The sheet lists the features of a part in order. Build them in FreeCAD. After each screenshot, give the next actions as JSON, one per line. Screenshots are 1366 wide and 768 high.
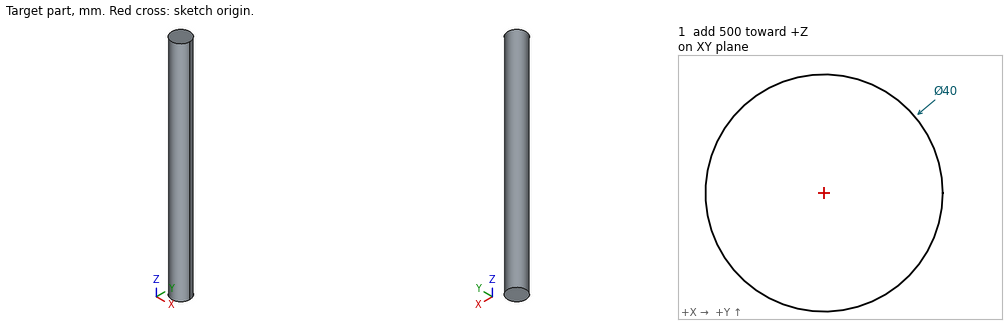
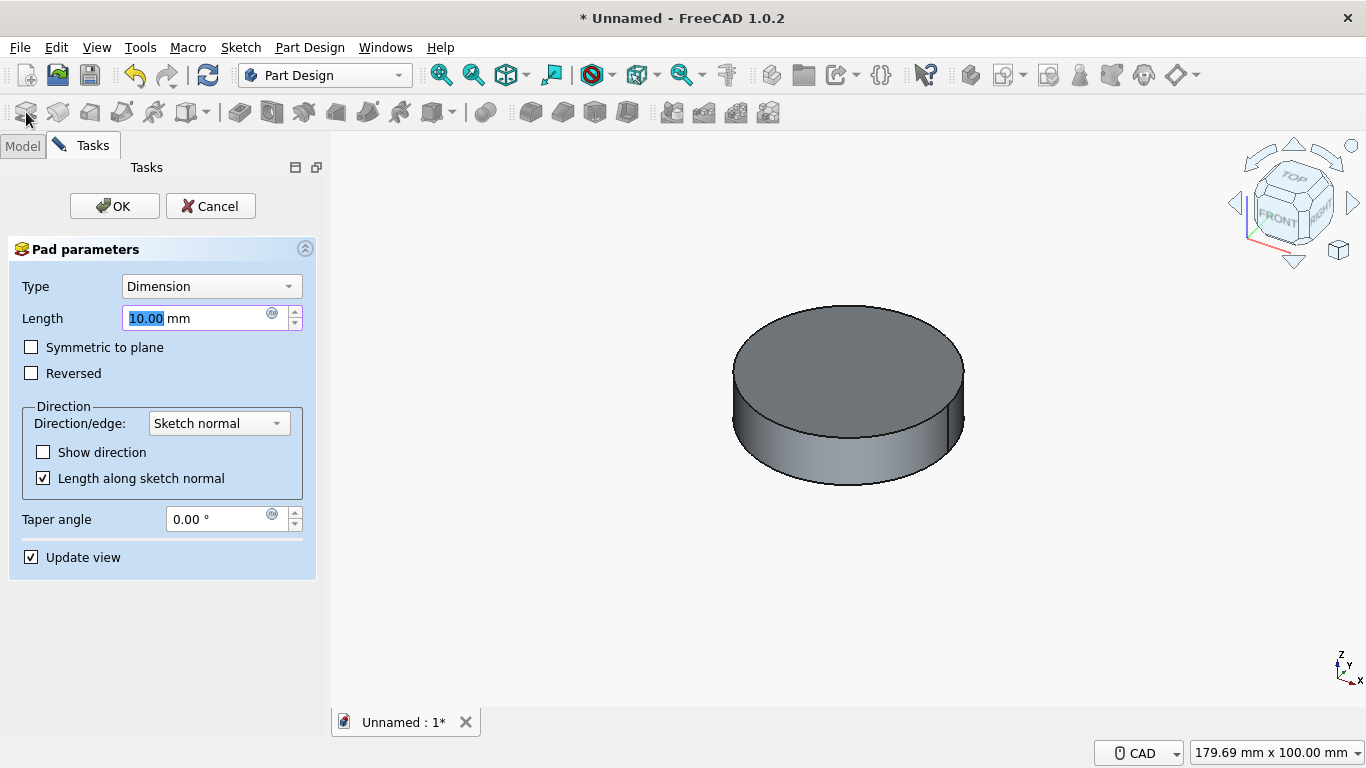
{"action": "type", "text": "500"}
{"action": "key", "text": "Tab"}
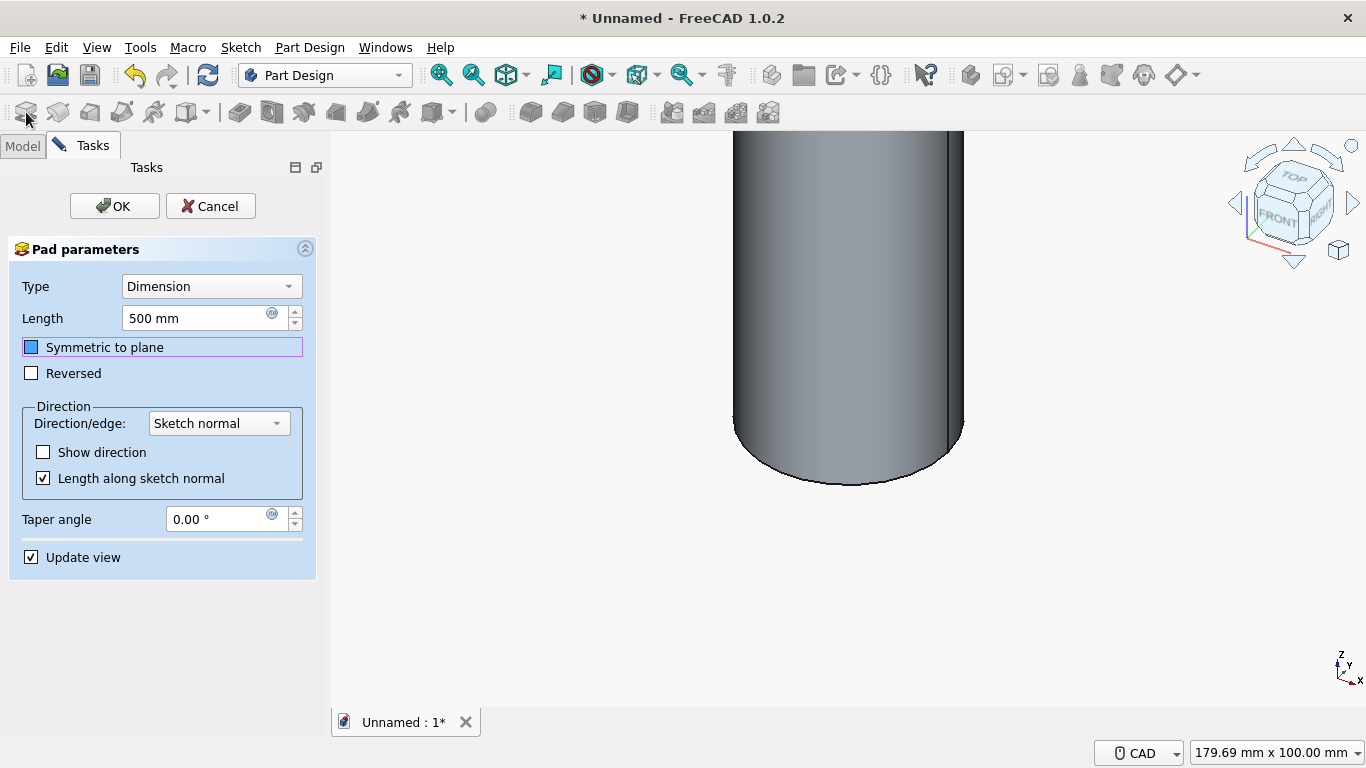
{"action": "left_click", "coordinate": [115, 206]}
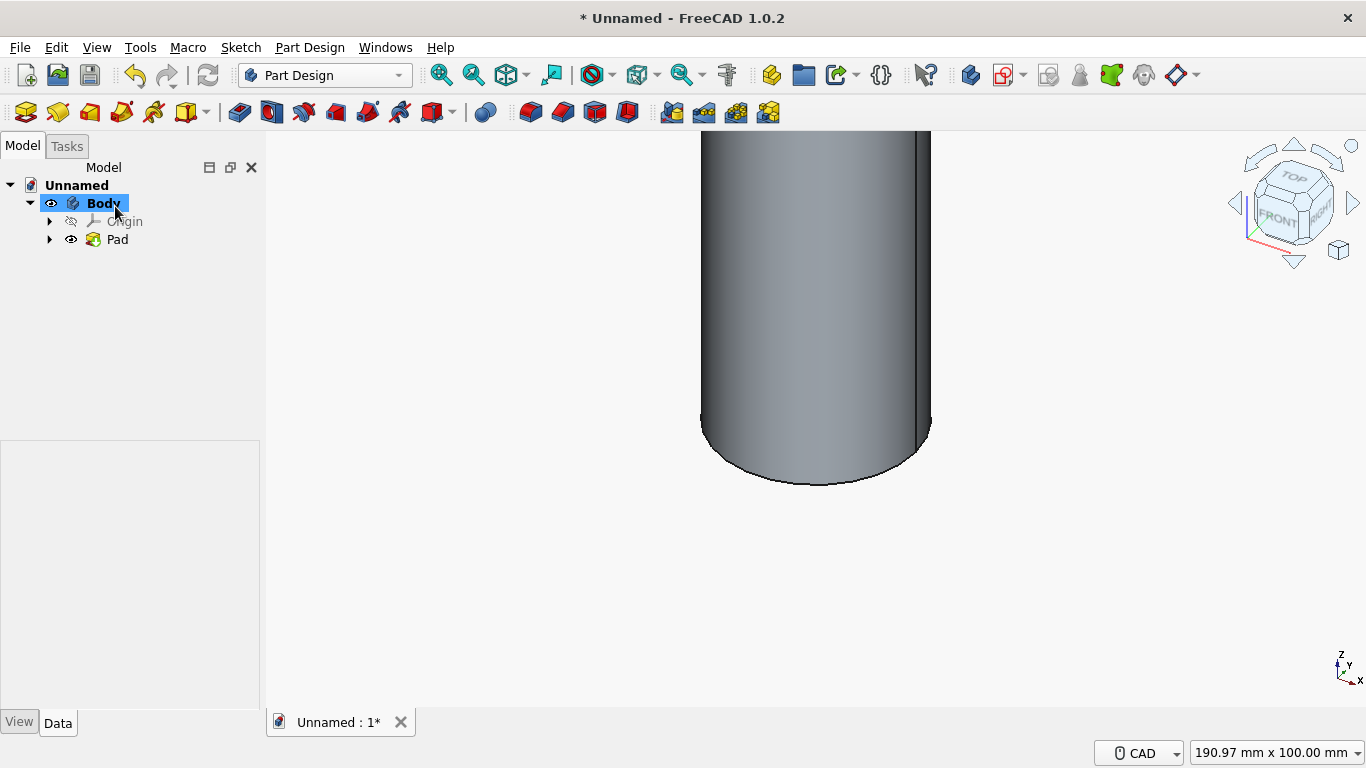
{"action": "key", "text": "0"}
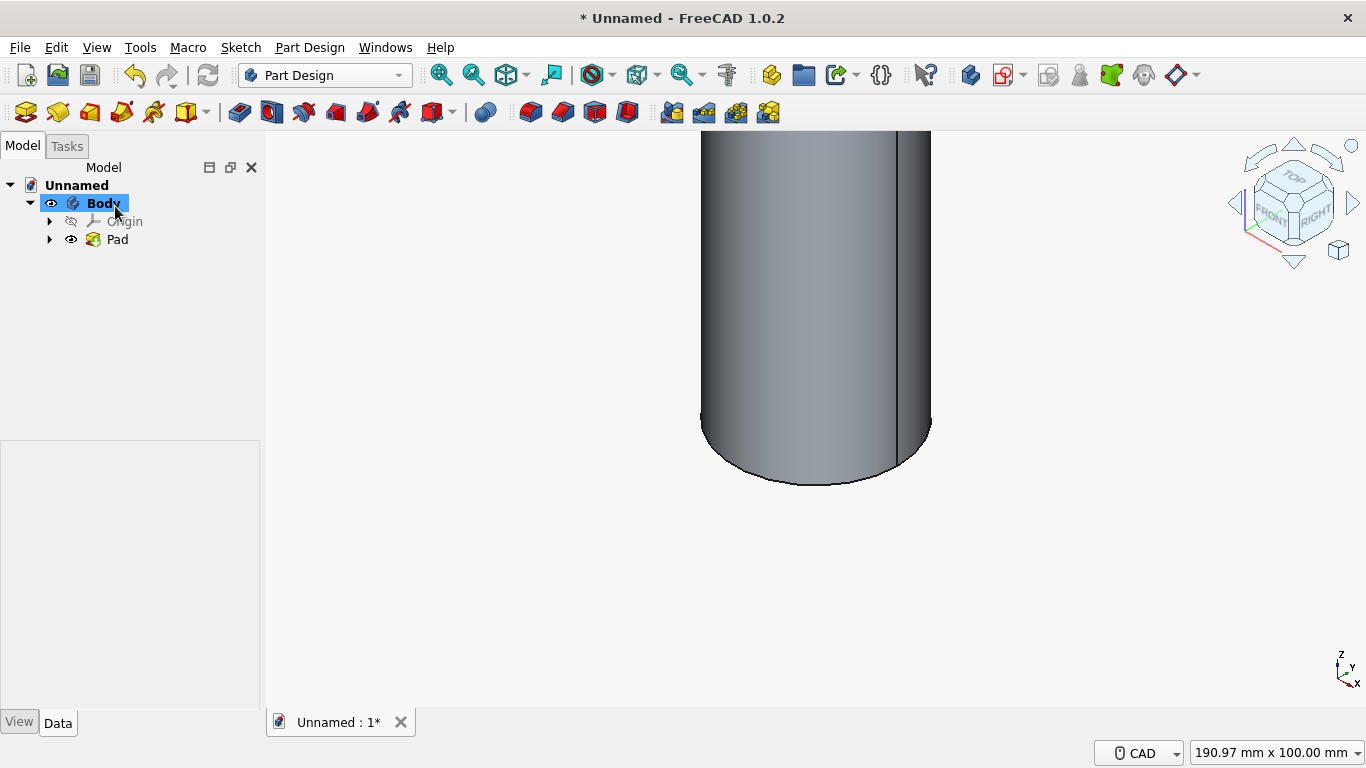
{"action": "left_click", "coordinate": [442, 76]}